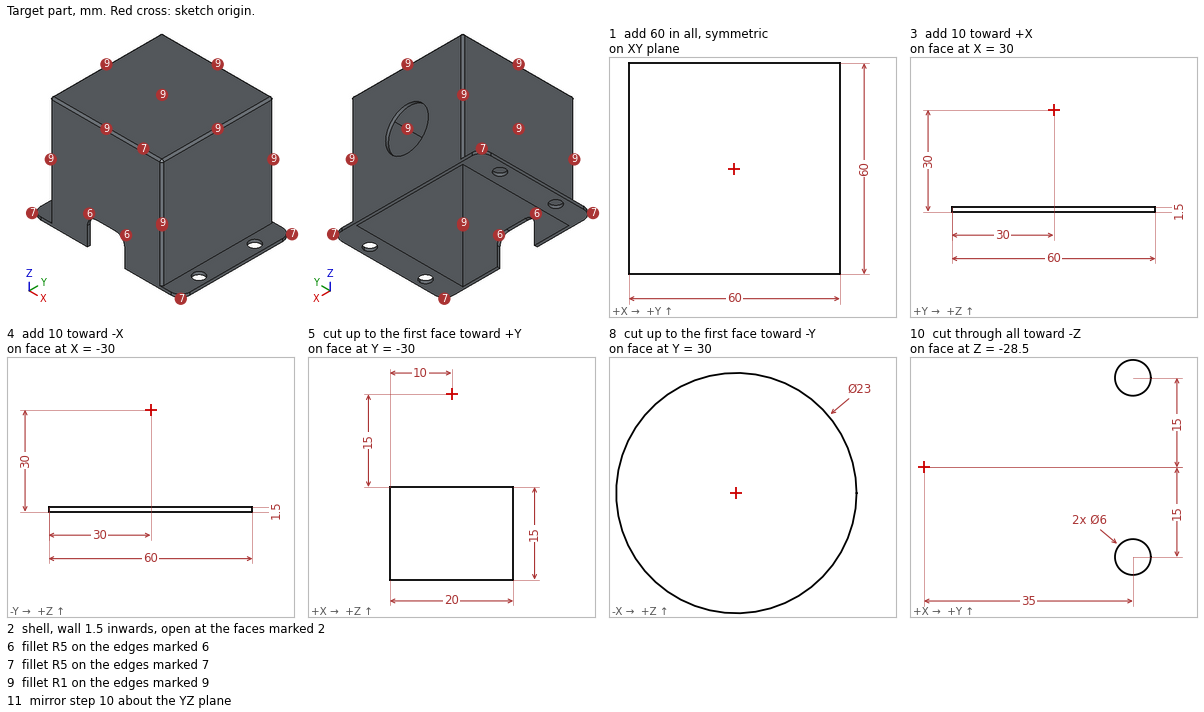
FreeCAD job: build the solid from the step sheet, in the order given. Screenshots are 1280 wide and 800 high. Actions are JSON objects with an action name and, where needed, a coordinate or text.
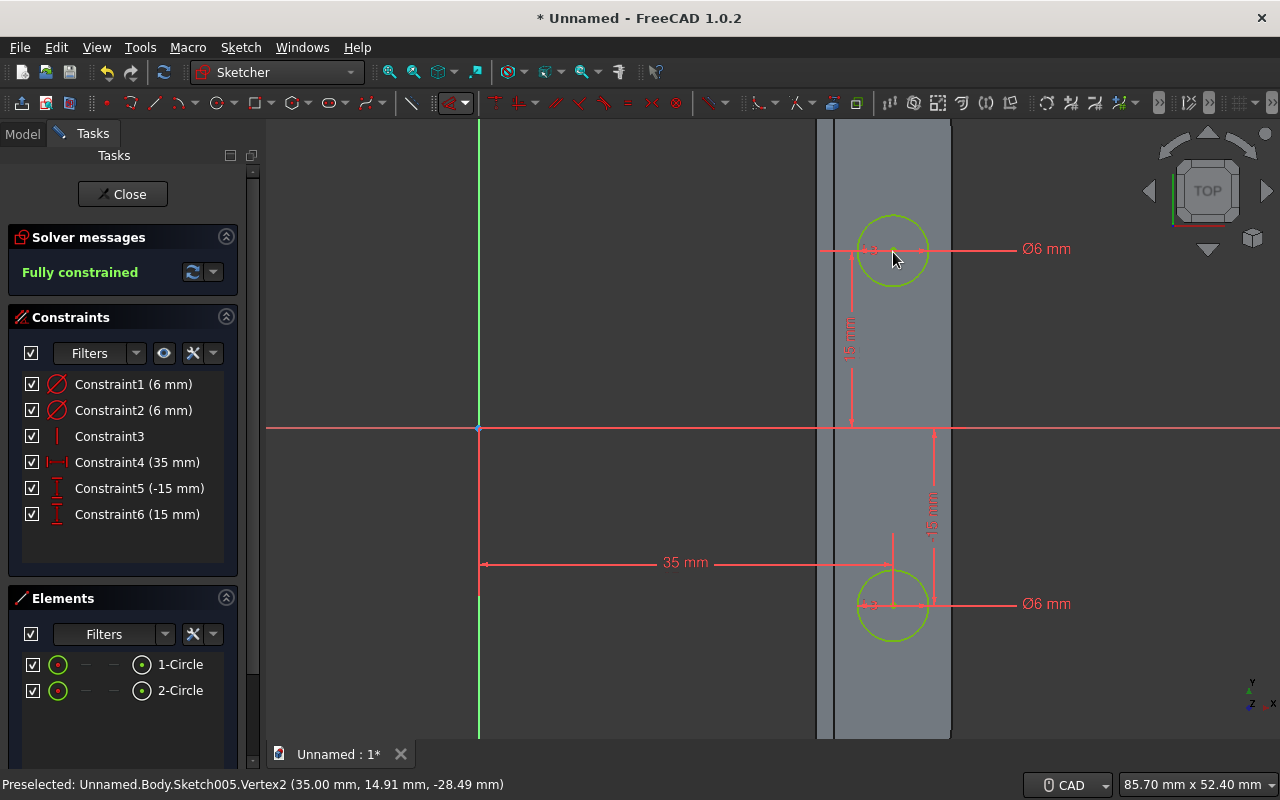
{"action": "left_click", "coordinate": [123, 194]}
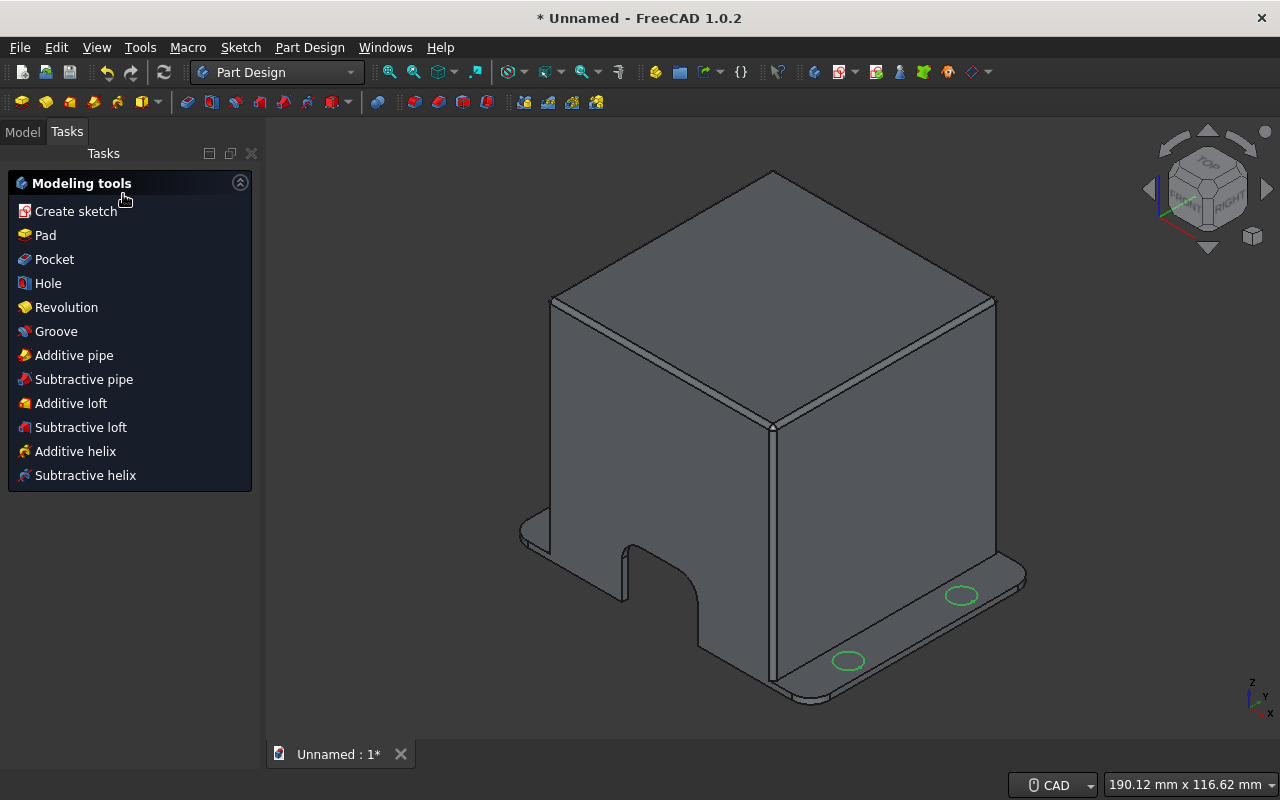
{"action": "left_click", "coordinate": [188, 102]}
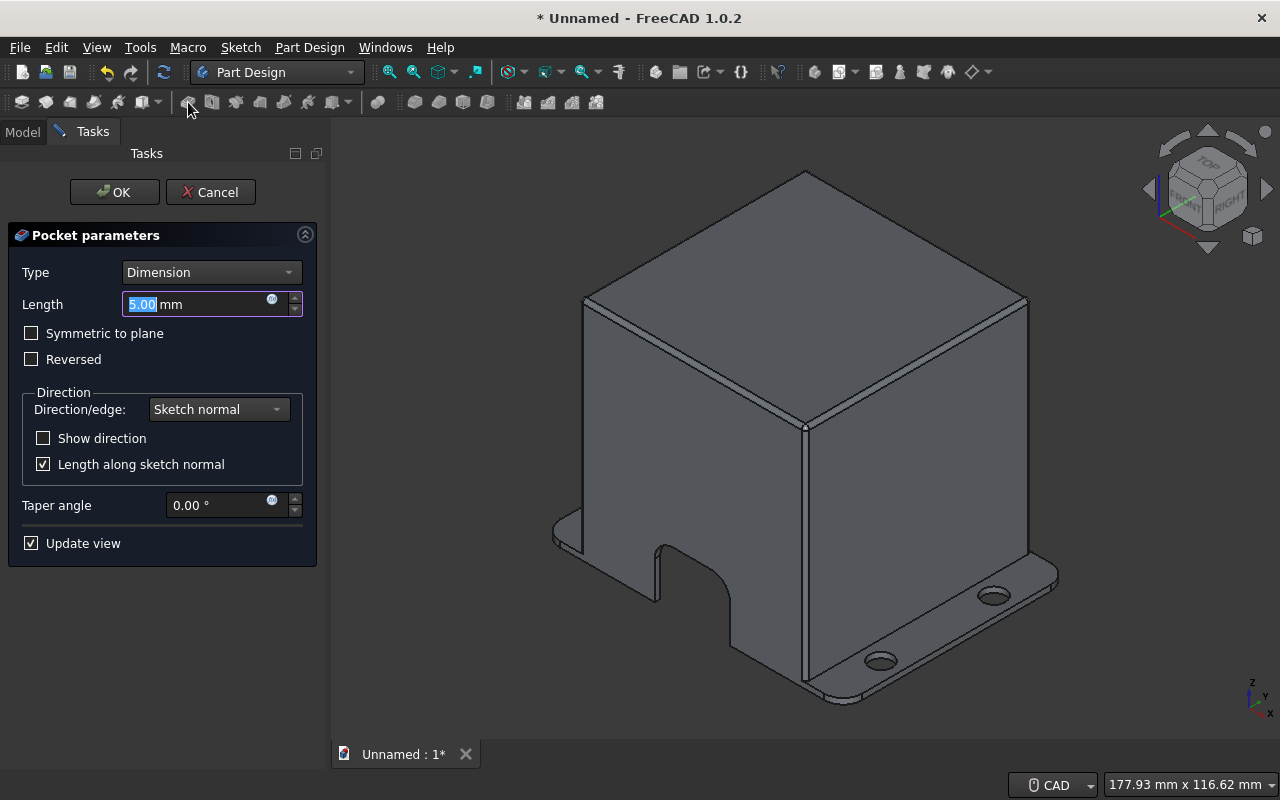
{"action": "left_click", "coordinate": [212, 272]}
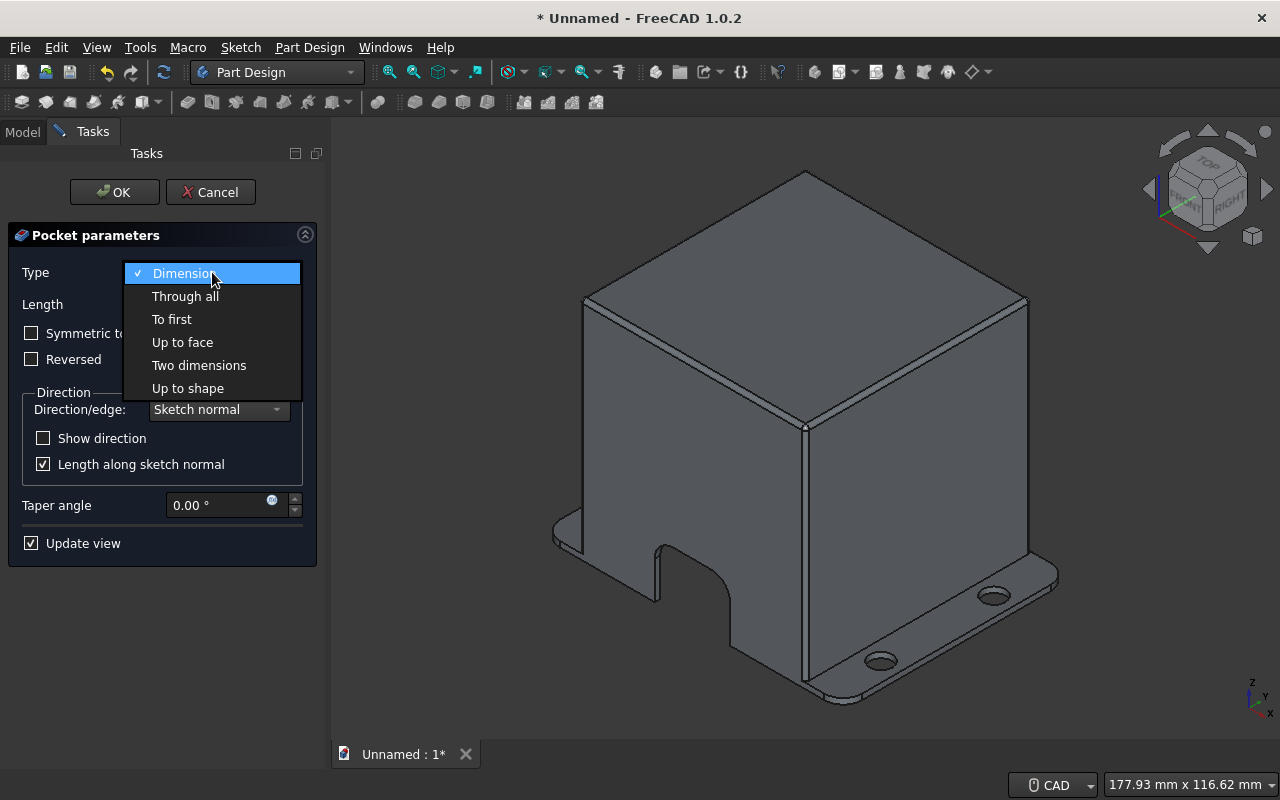
{"action": "left_click", "coordinate": [212, 296]}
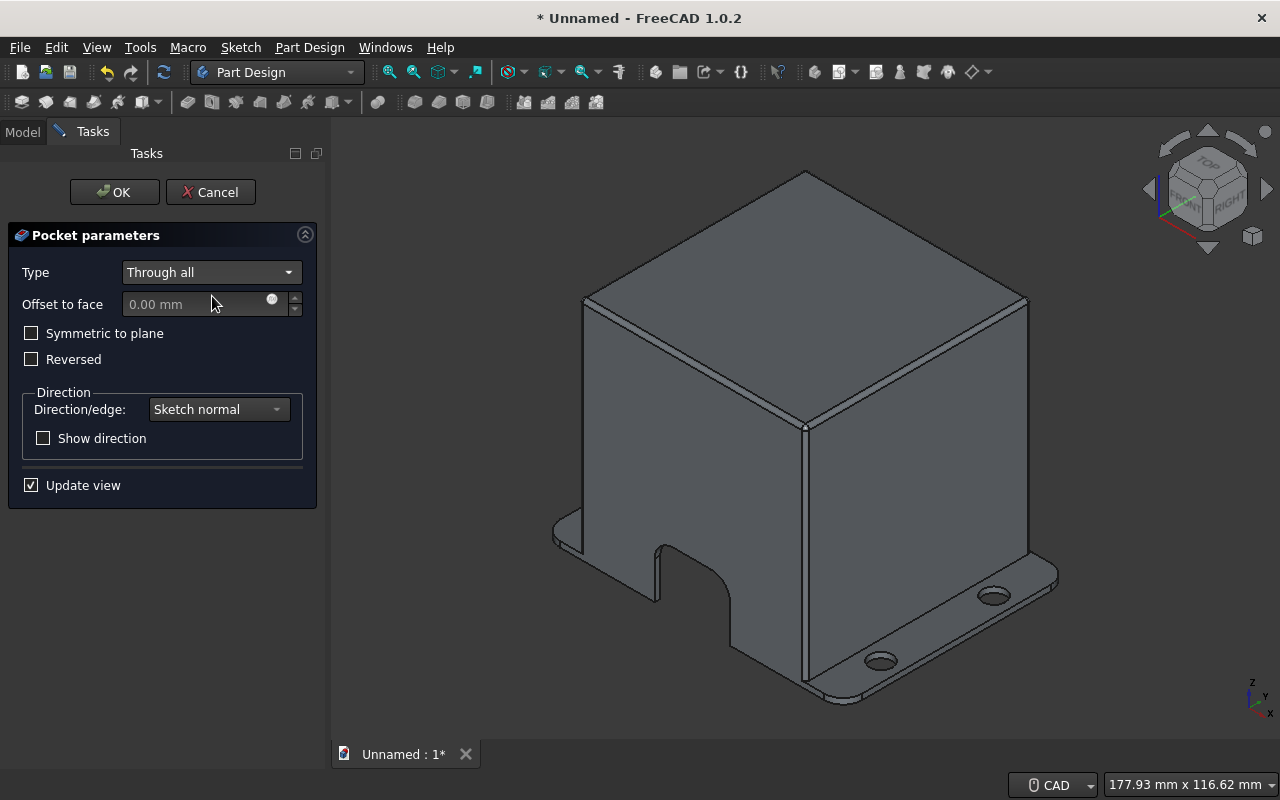
{"action": "left_click", "coordinate": [115, 192]}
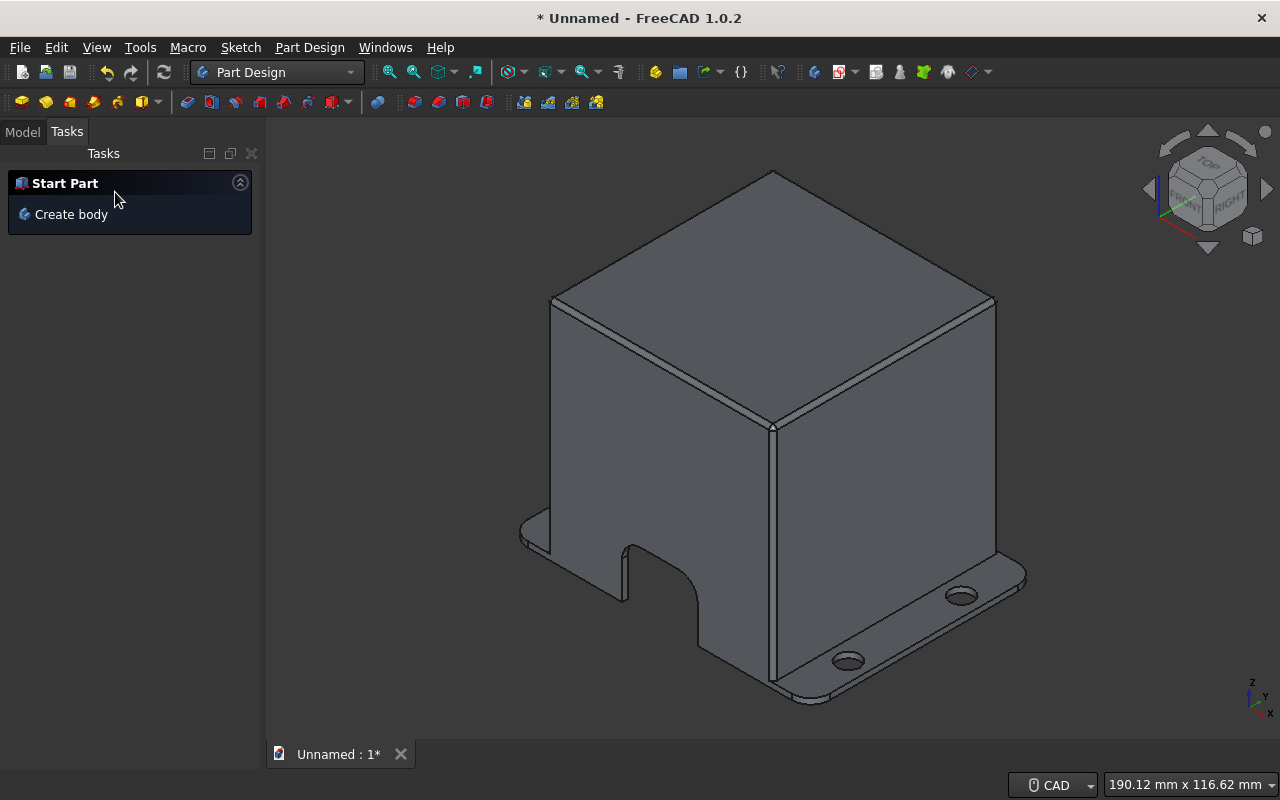
{"action": "left_click", "coordinate": [23, 131]}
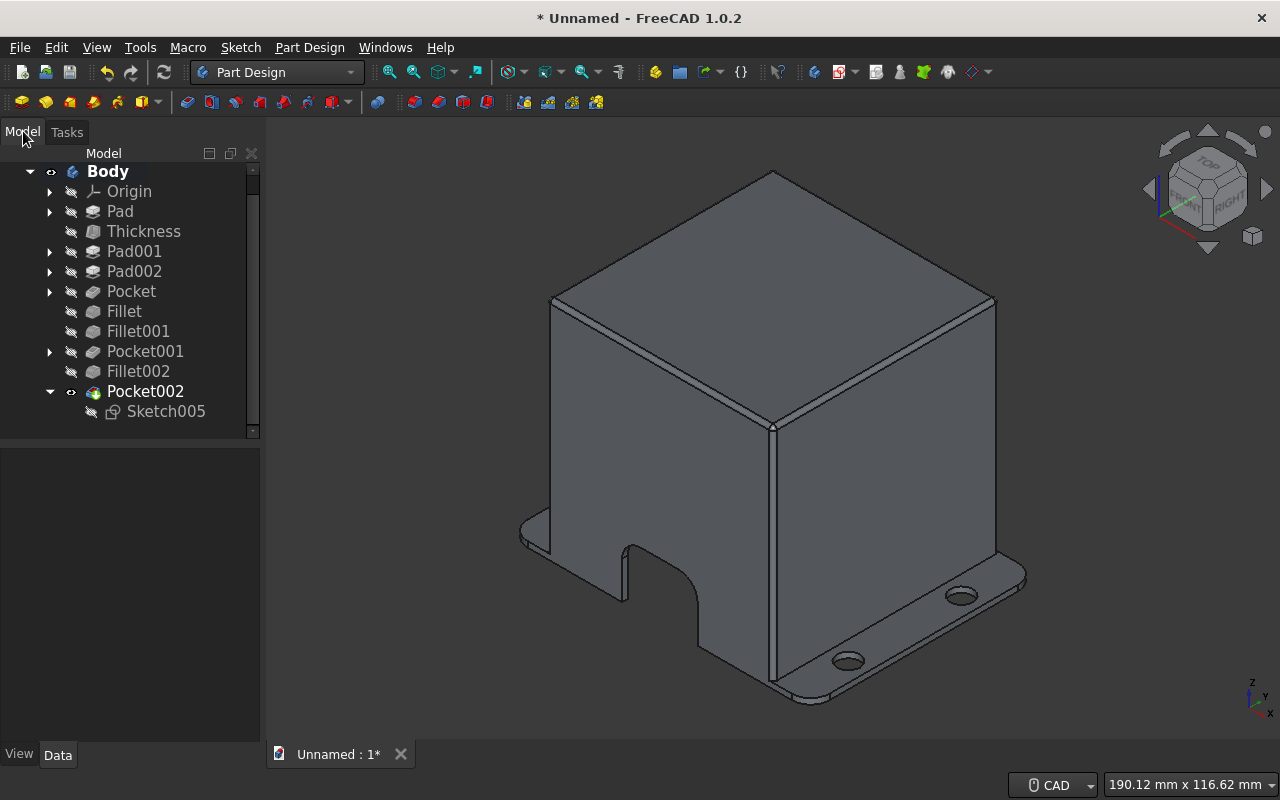
{"action": "left_click", "coordinate": [116, 392]}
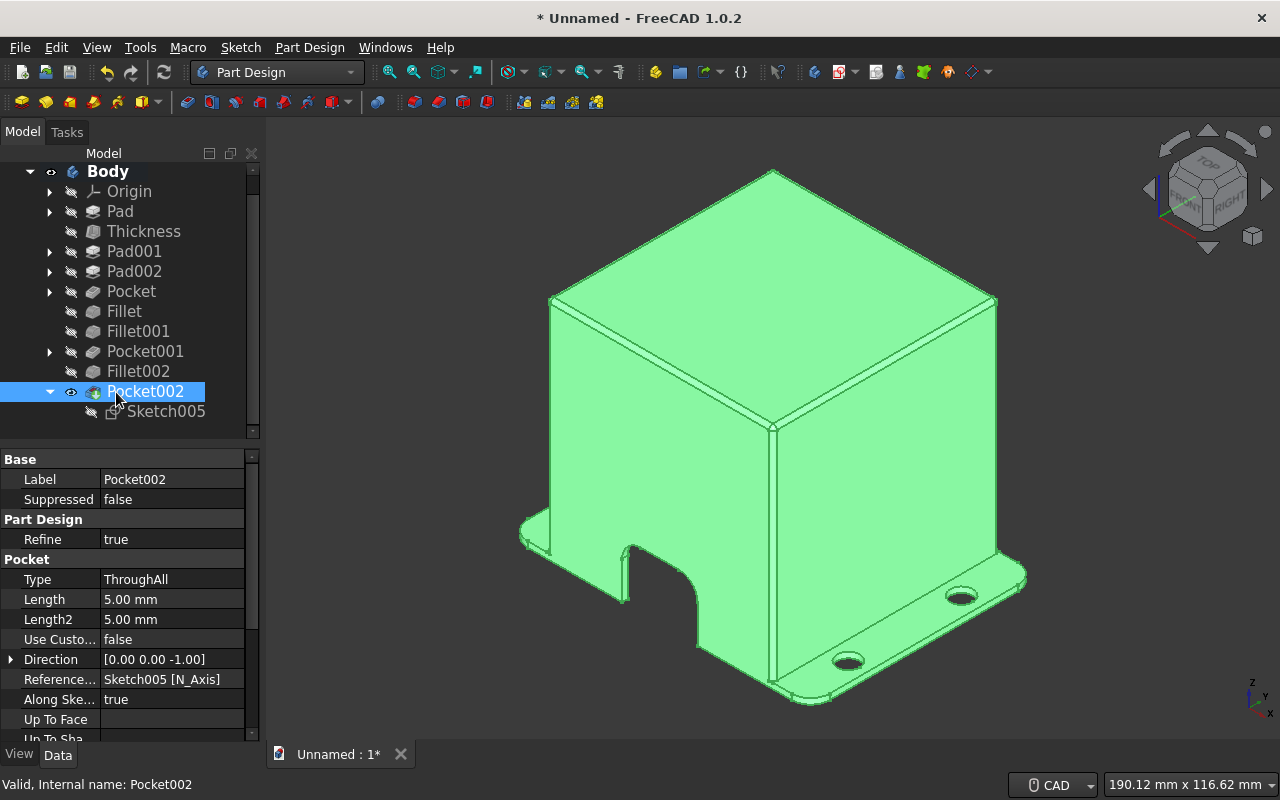
{"action": "left_click", "coordinate": [524, 102]}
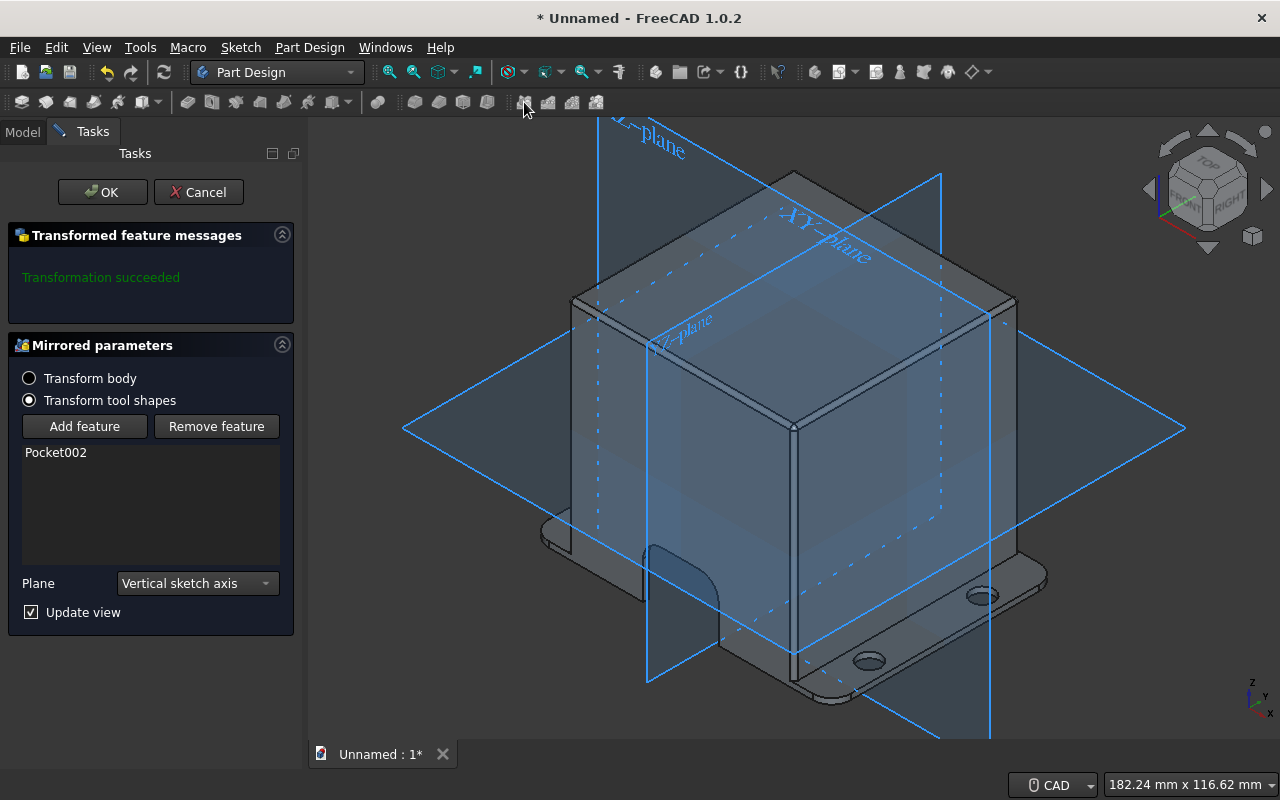
{"action": "left_click", "coordinate": [198, 584]}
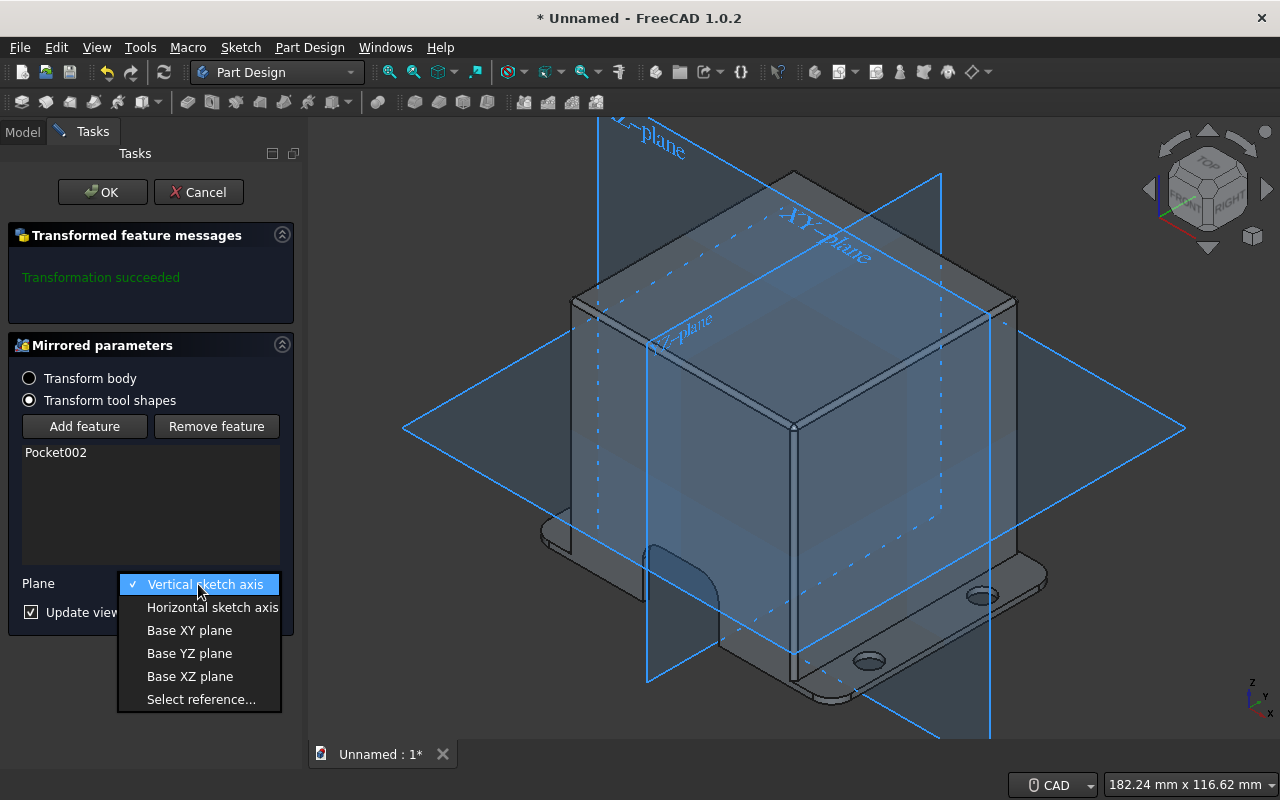
{"action": "left_click", "coordinate": [198, 654]}